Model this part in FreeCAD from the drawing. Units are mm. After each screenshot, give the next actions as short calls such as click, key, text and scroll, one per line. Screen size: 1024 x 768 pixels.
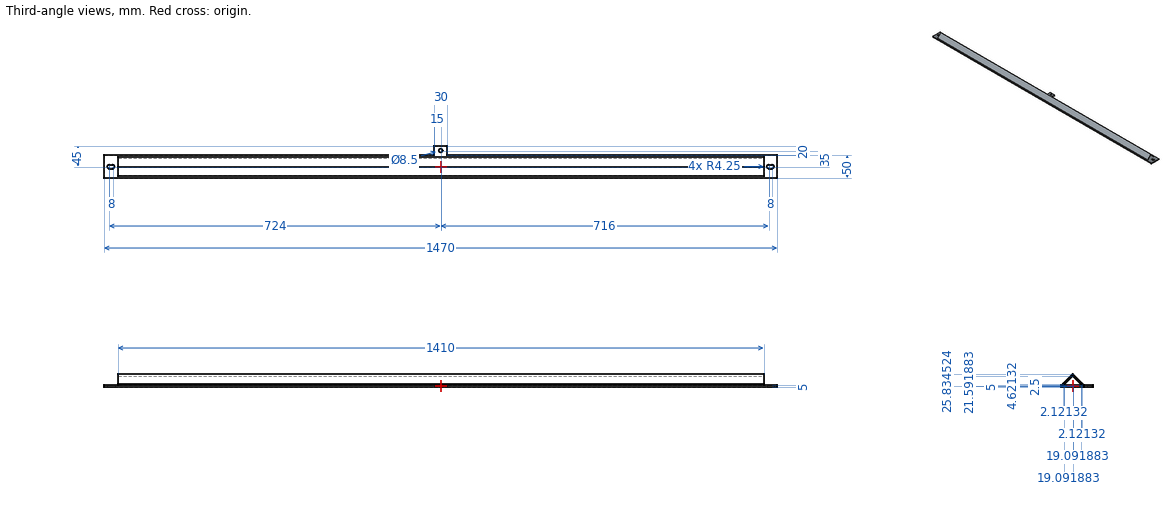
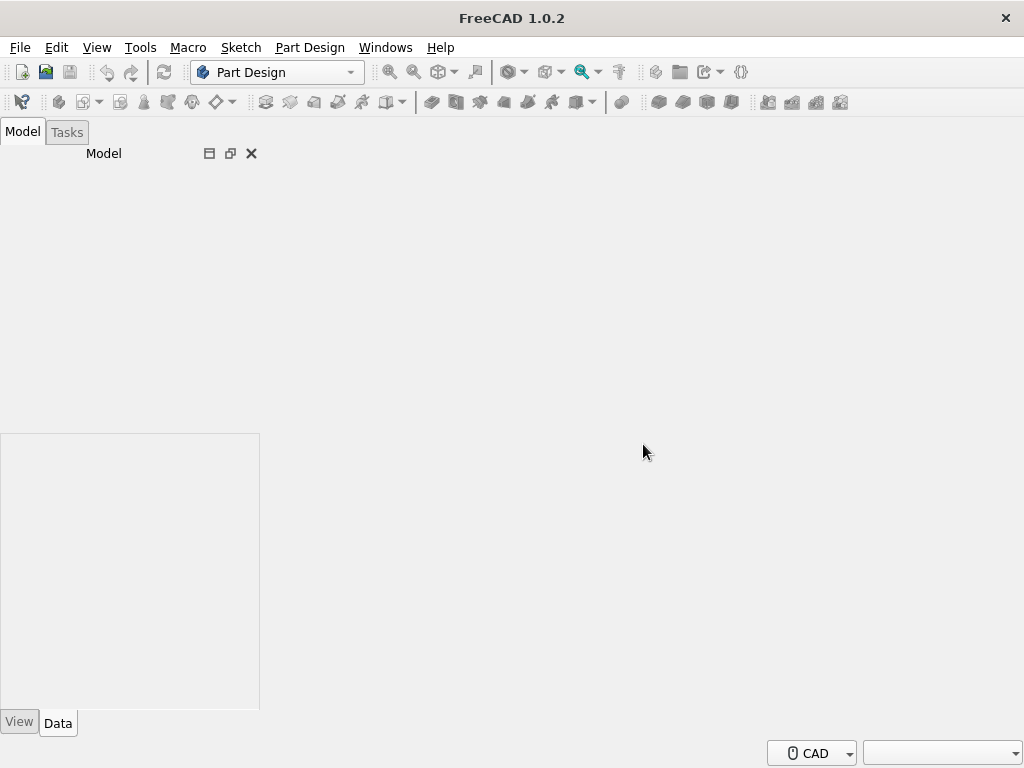
click(22, 72)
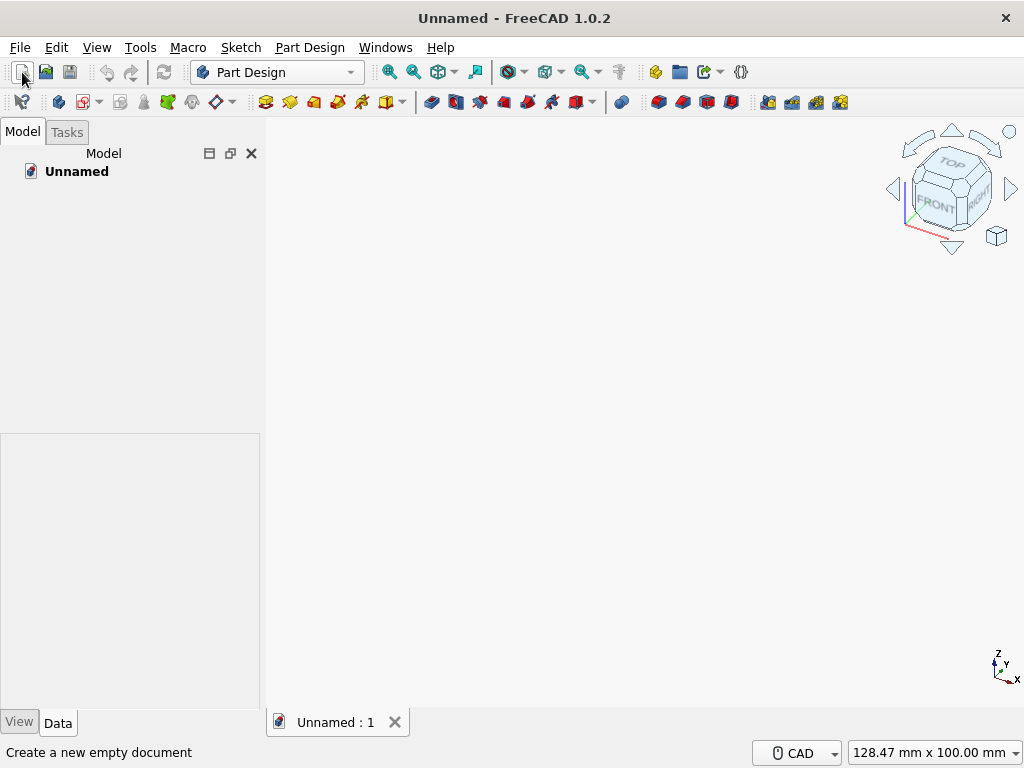
click(84, 102)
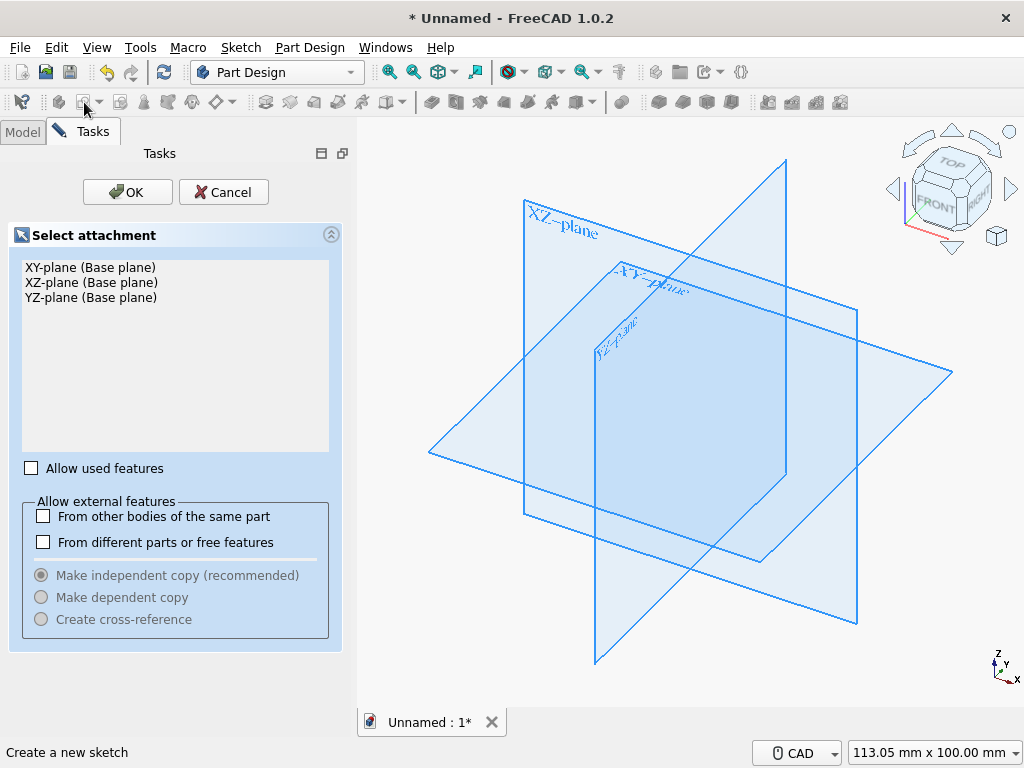
click(82, 268)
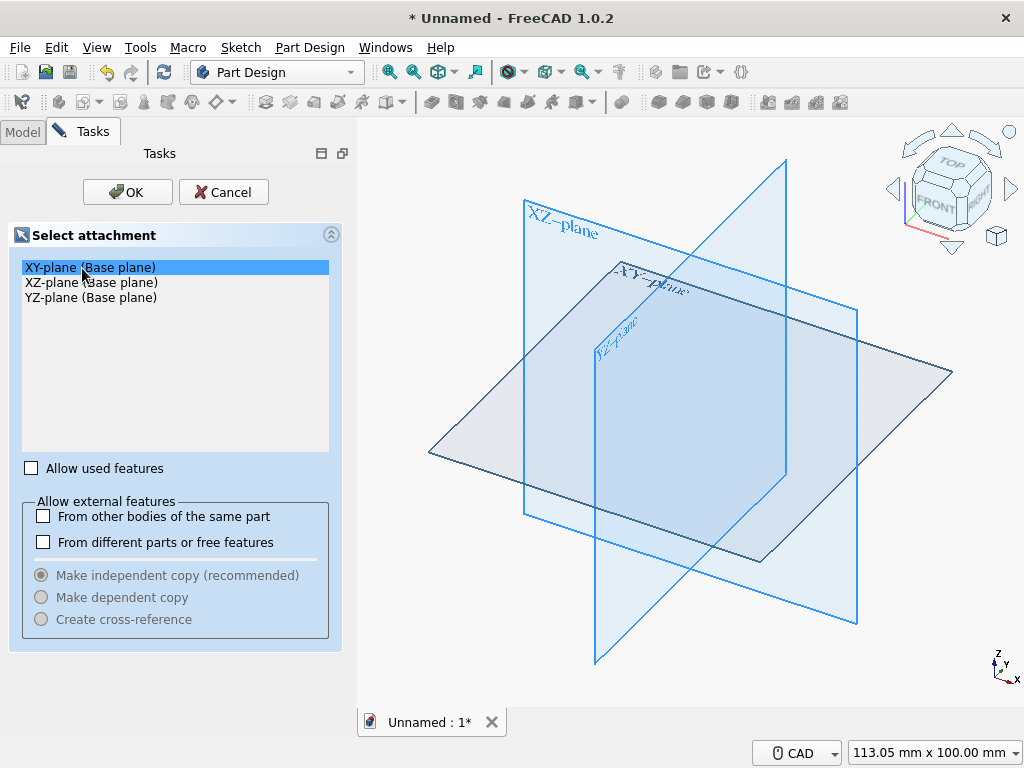
click(128, 192)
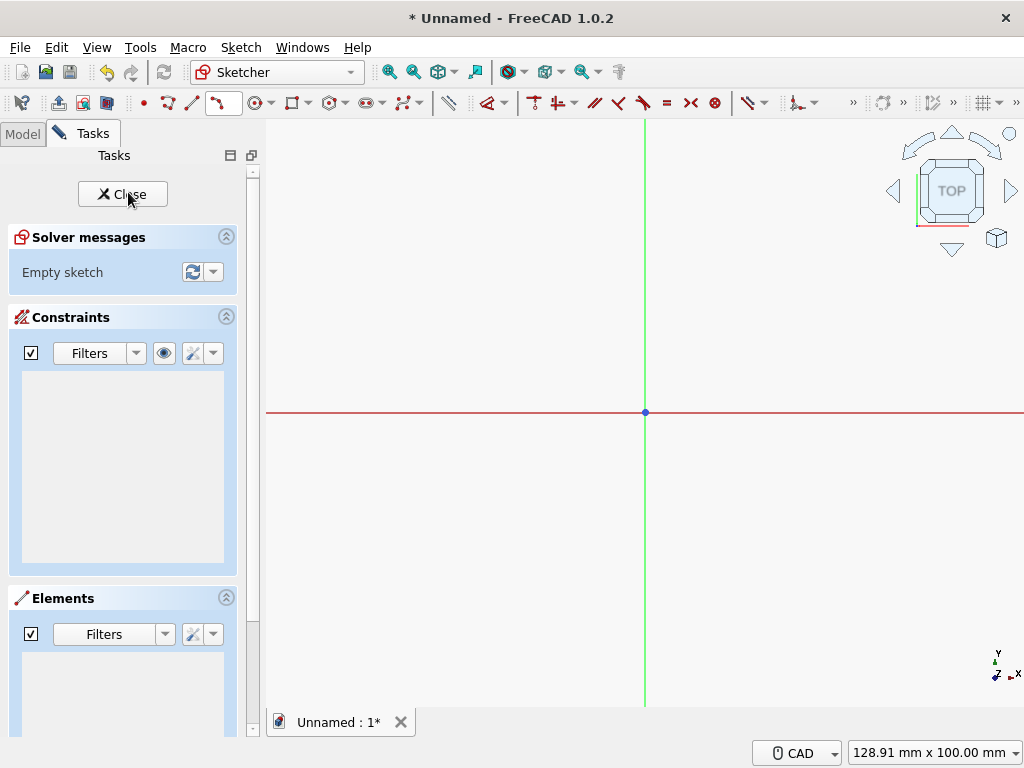
scroll(573, 413, down, 15)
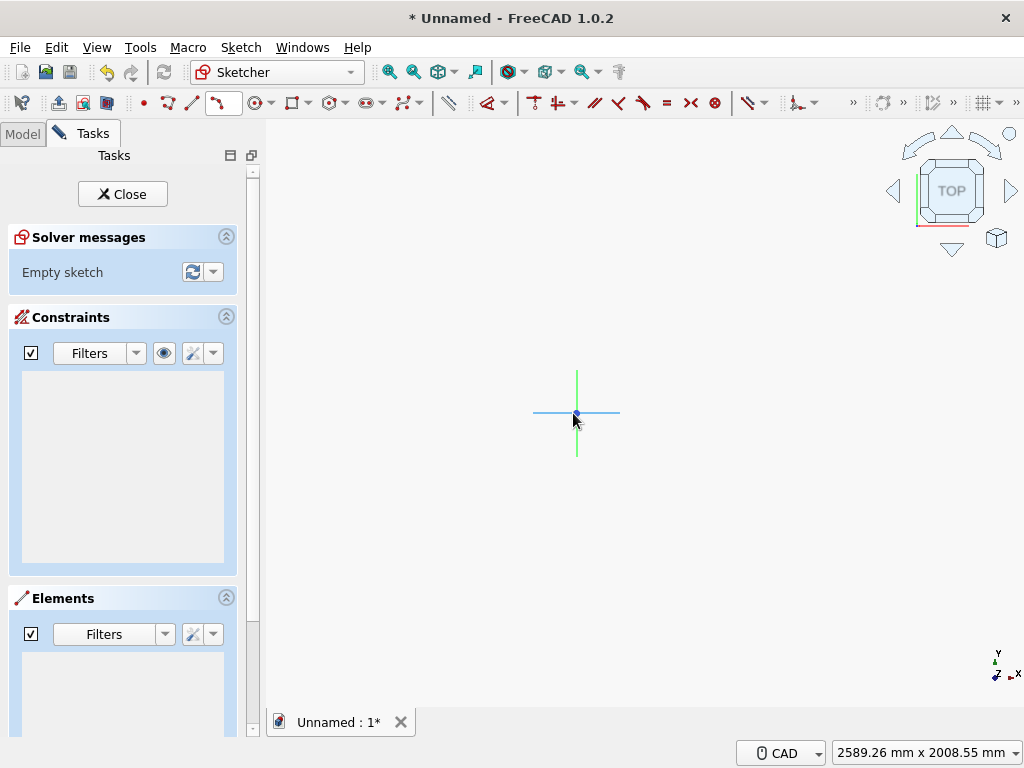
key(g)
key(v)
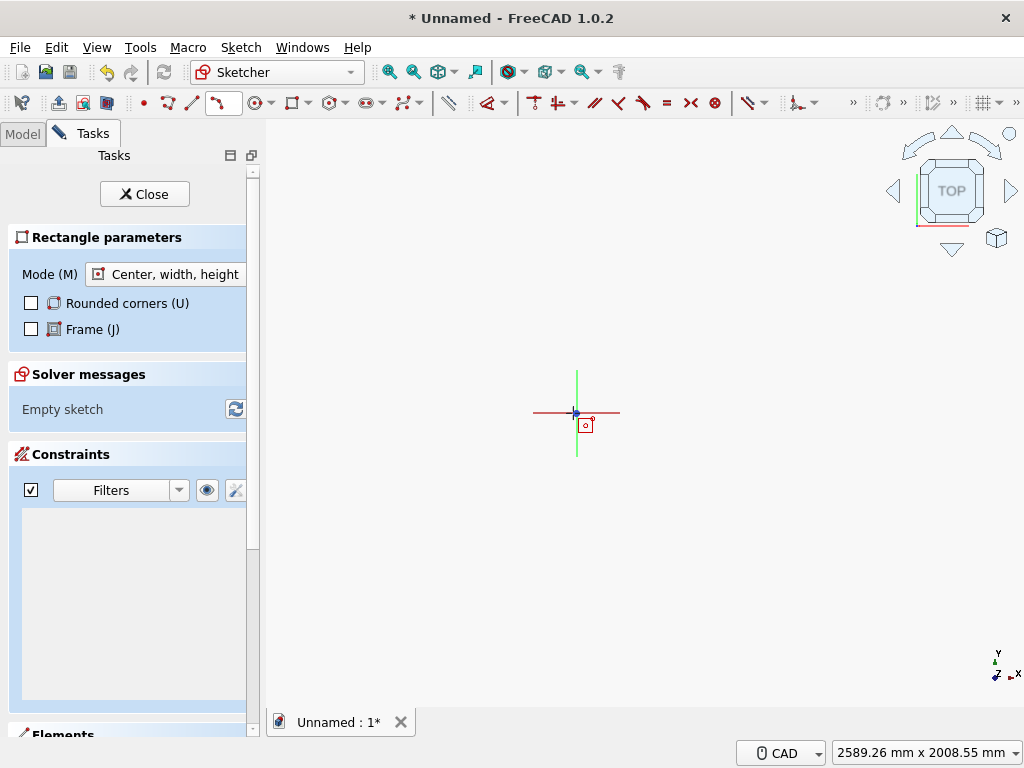
scroll(577, 413, up, 4)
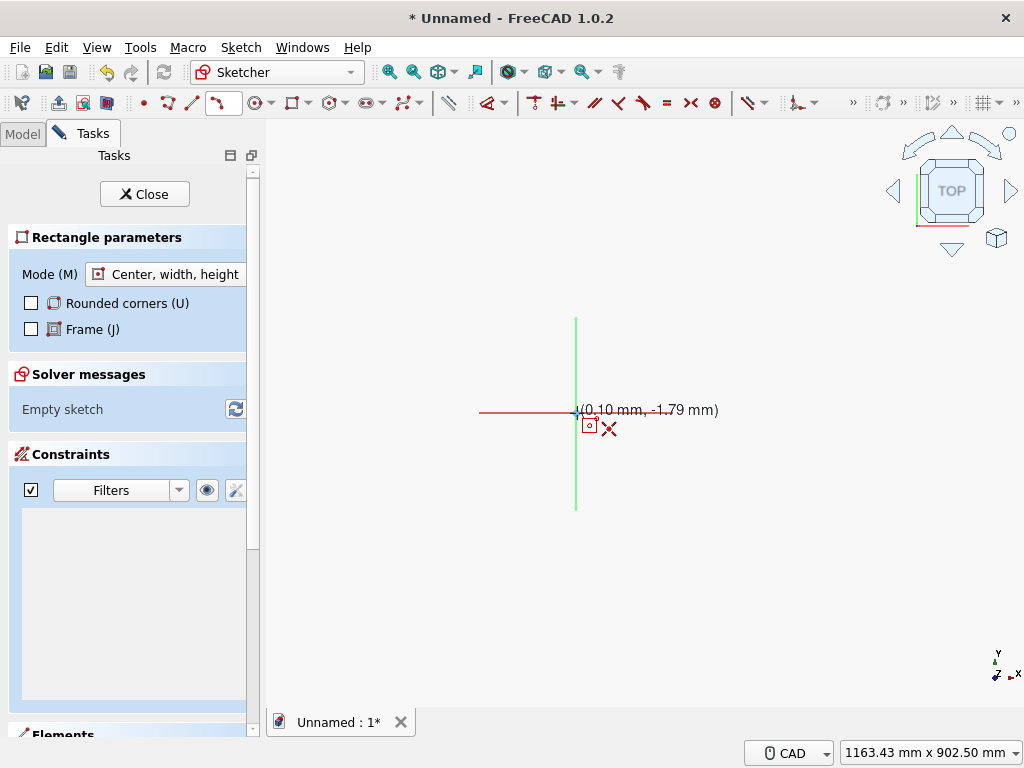
click(576, 413)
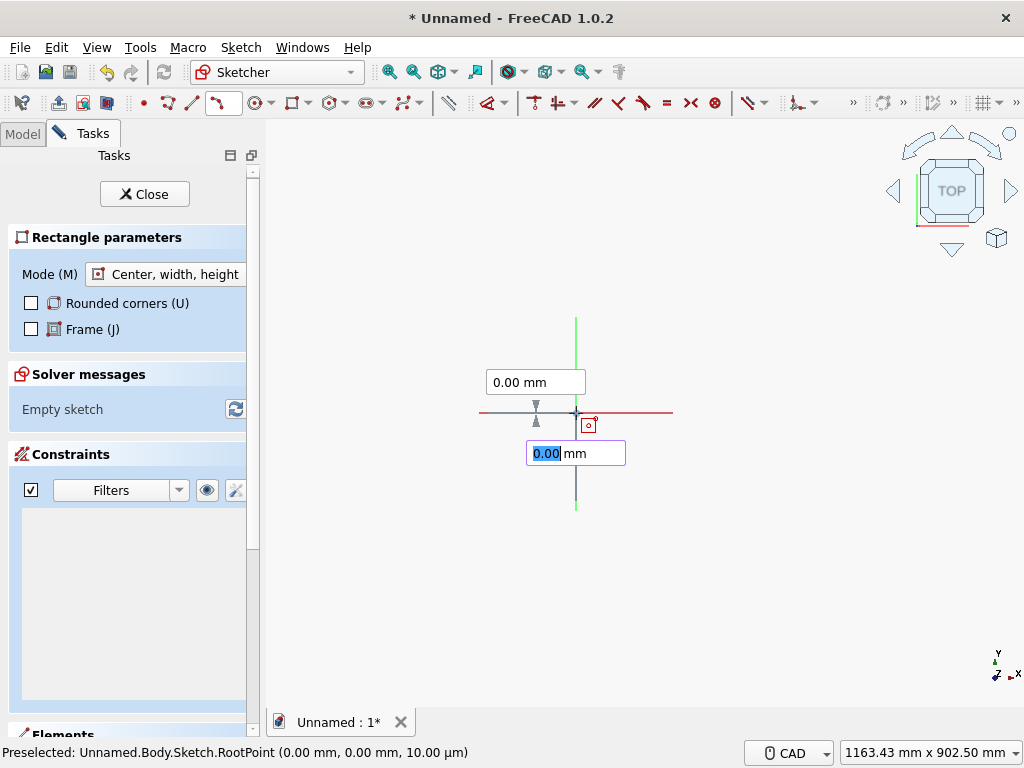
scroll(577, 413, down, 4)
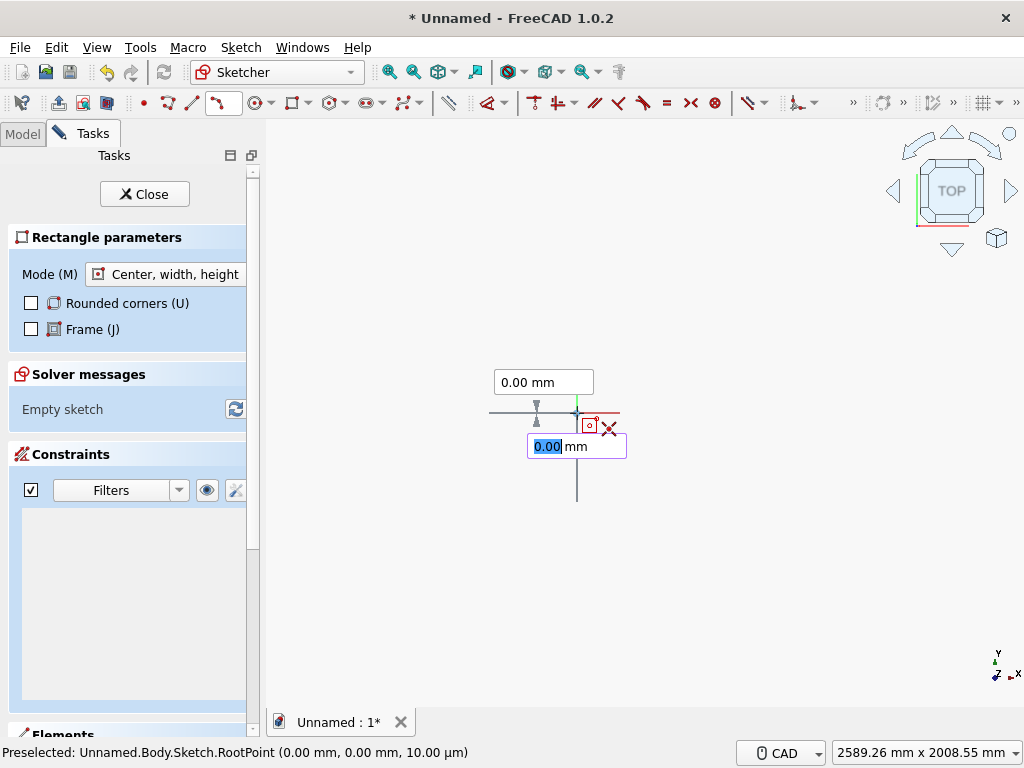
scroll(792, 406, up, 4)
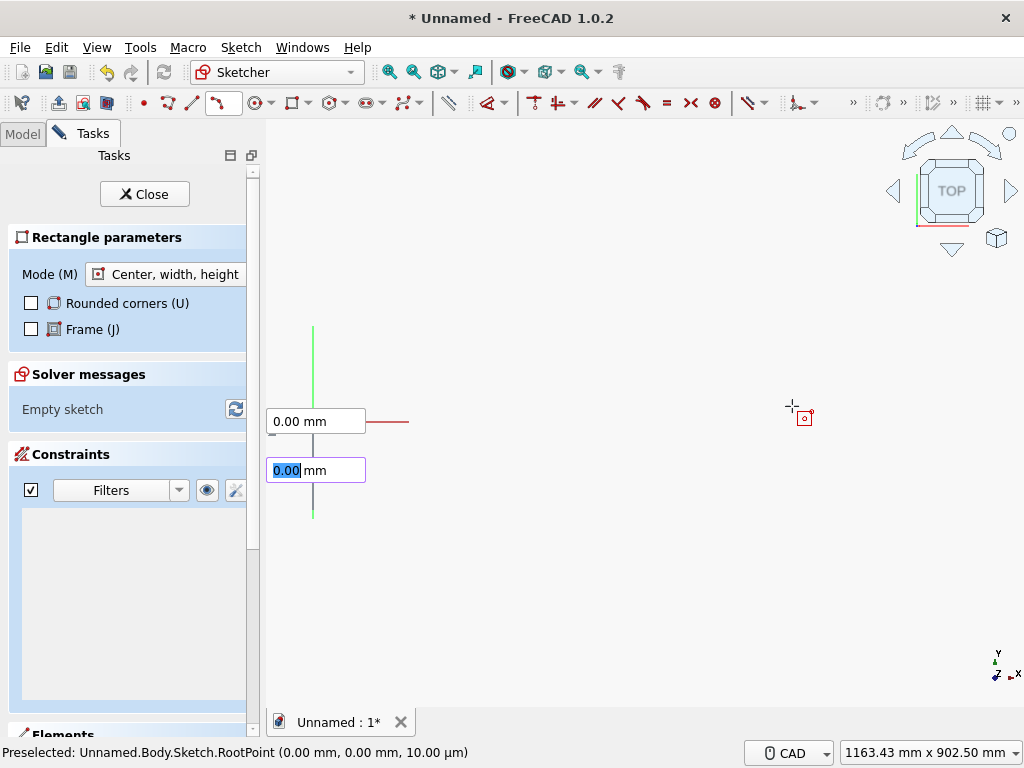
click(791, 406)
key(Escape)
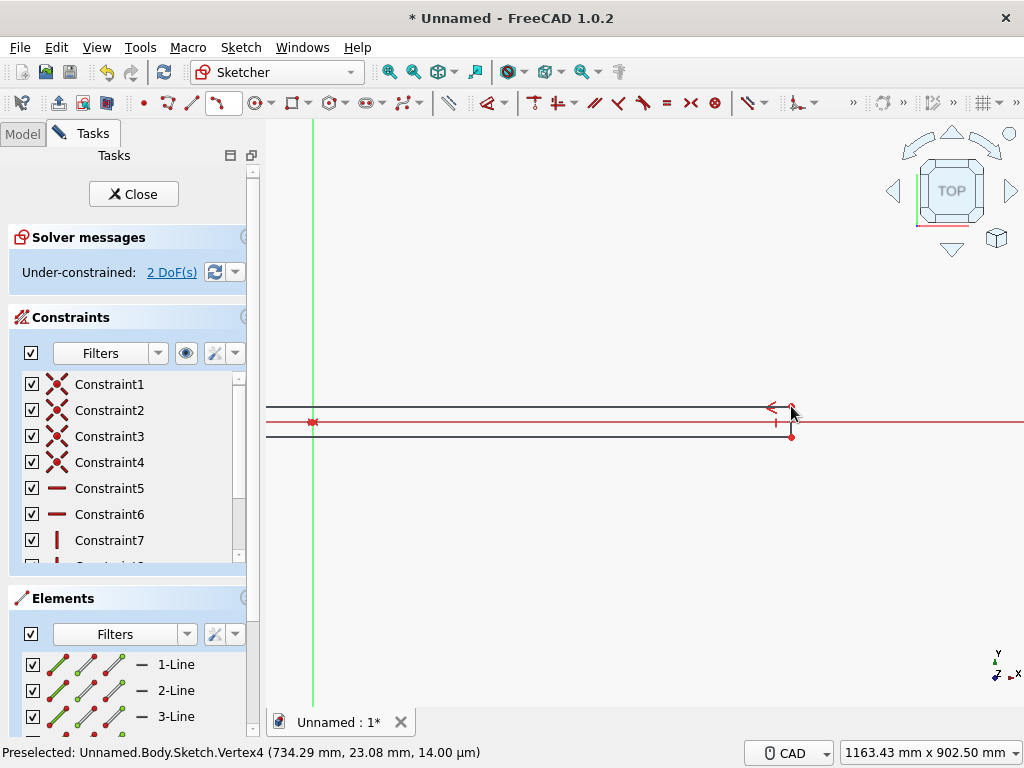
click(791, 425)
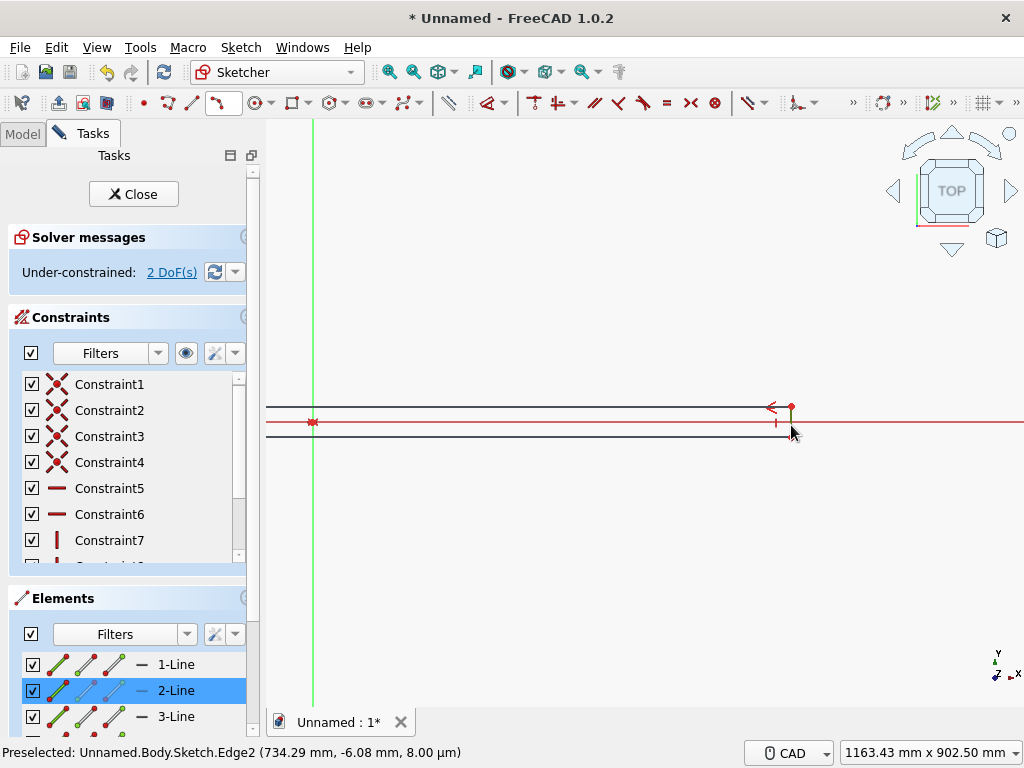
key(i)